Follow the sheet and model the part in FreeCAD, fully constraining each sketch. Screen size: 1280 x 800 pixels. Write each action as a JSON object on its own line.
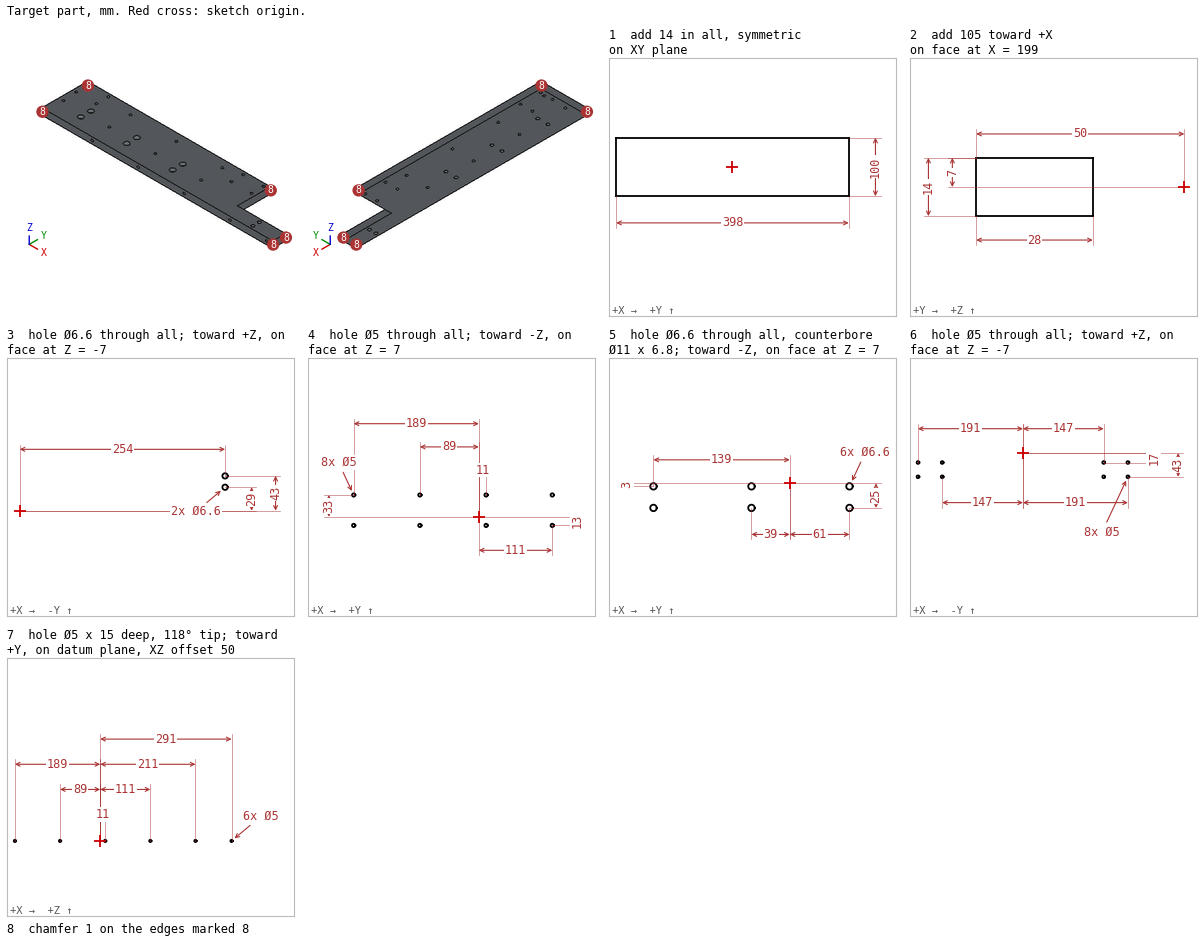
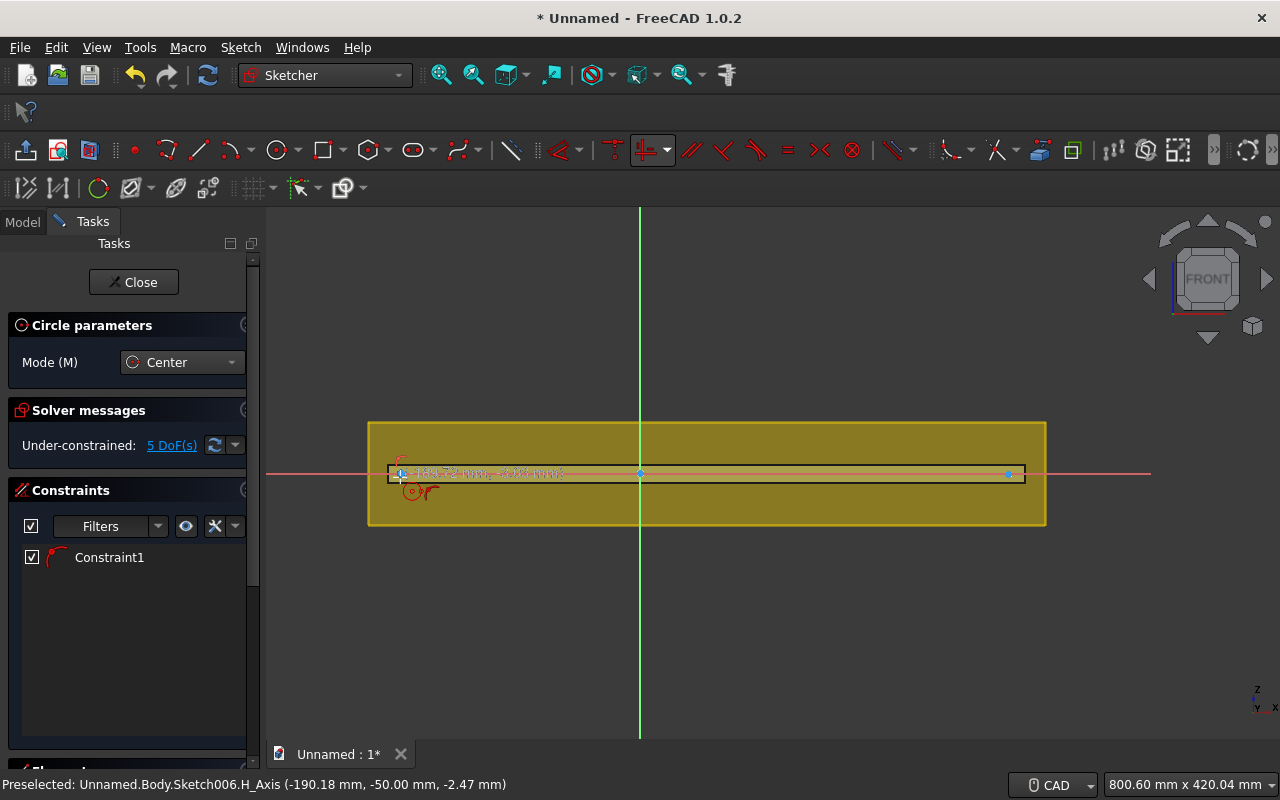
{"action": "scroll", "coordinate": [528, 474], "scroll_direction": "up", "scroll_amount": 10}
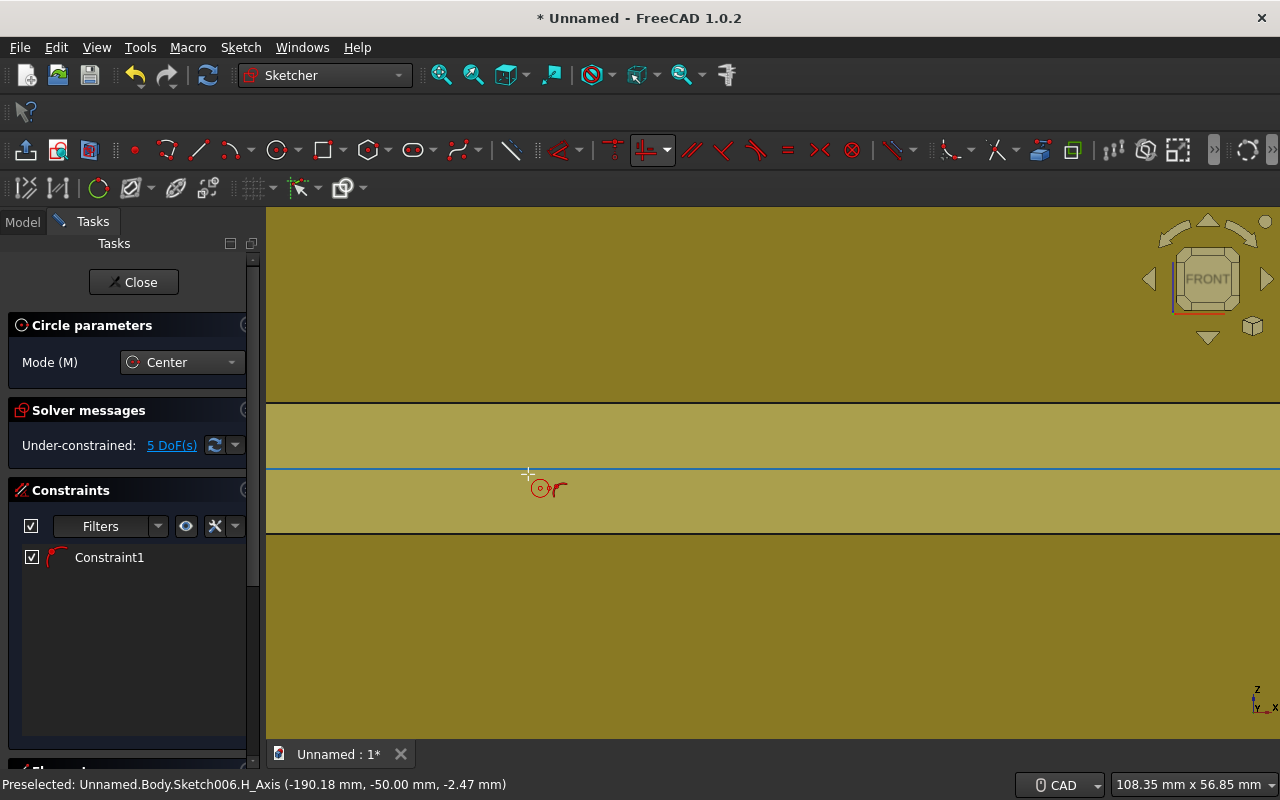
{"action": "scroll", "coordinate": [528, 474], "scroll_direction": "down", "scroll_amount": 10}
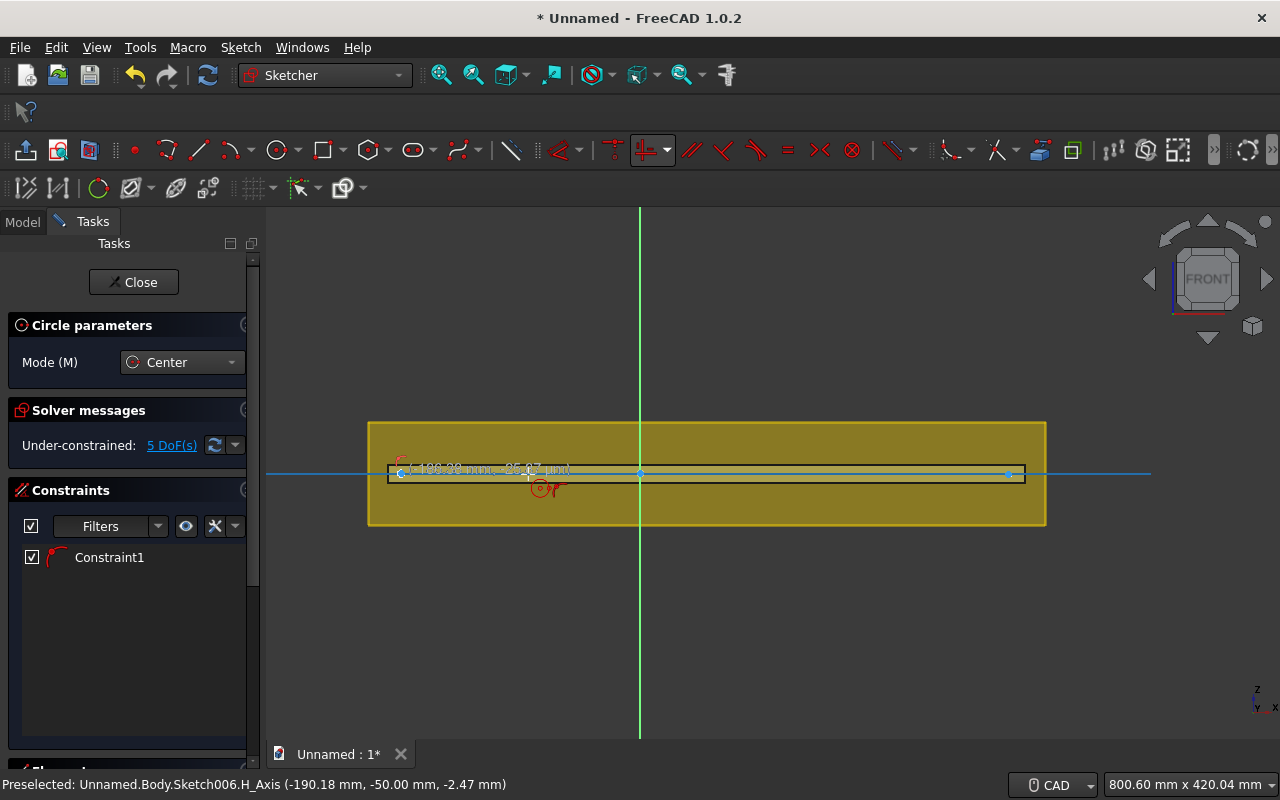
{"action": "left_click", "coordinate": [528, 474]}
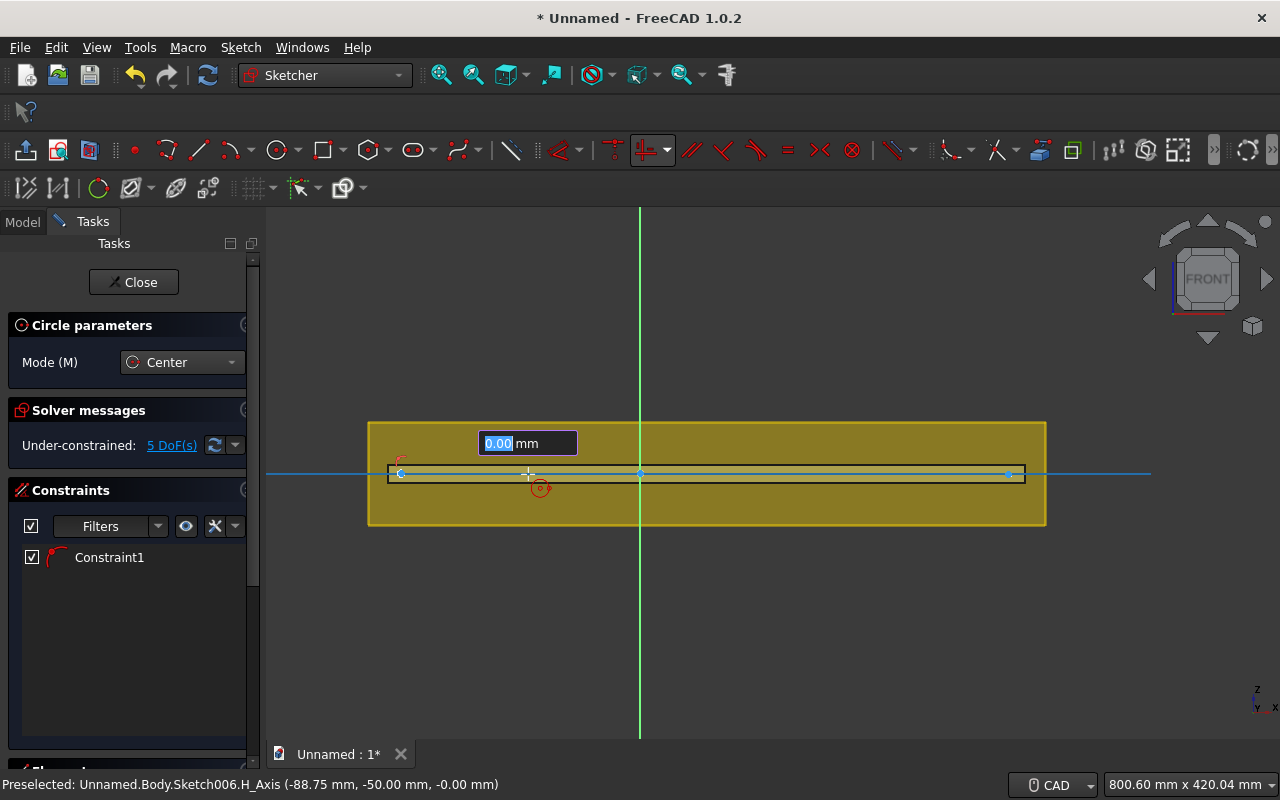
{"action": "scroll", "coordinate": [527, 477], "scroll_direction": "up", "scroll_amount": 9}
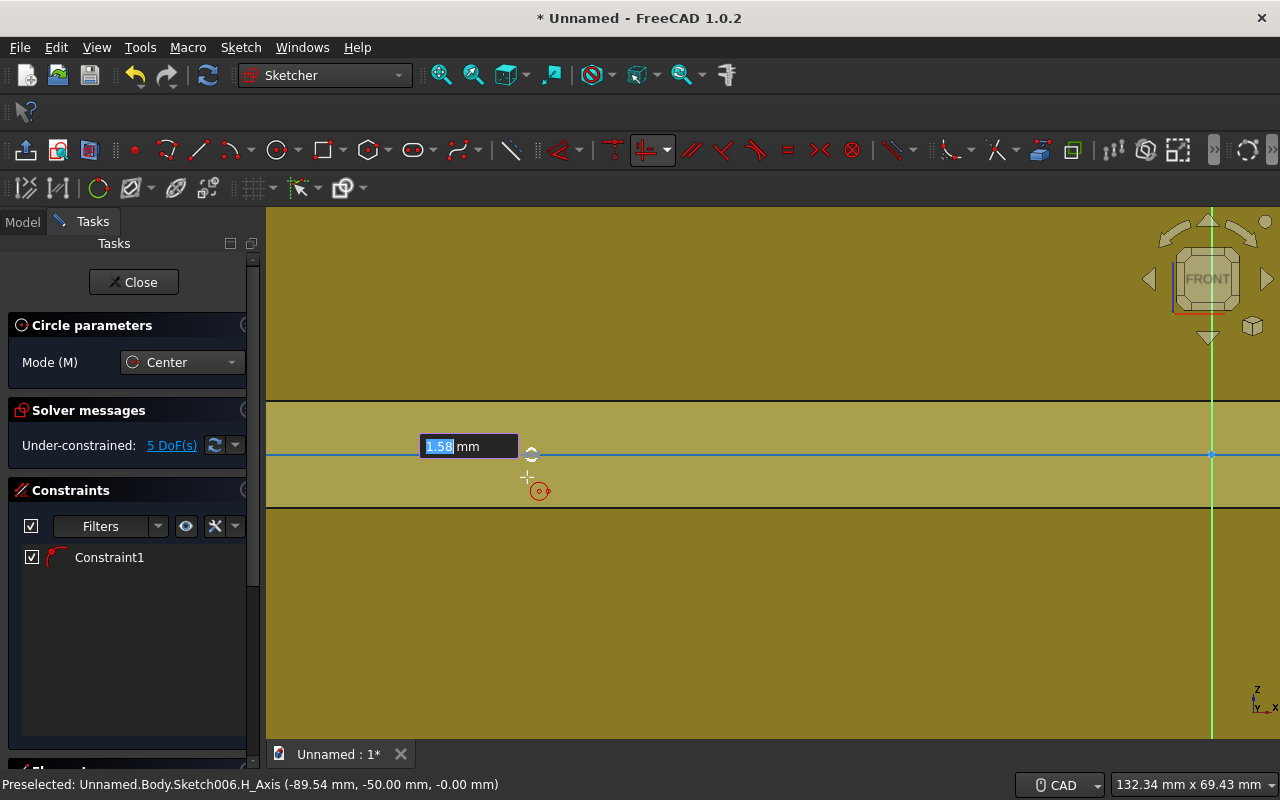
{"action": "left_click", "coordinate": [523, 473]}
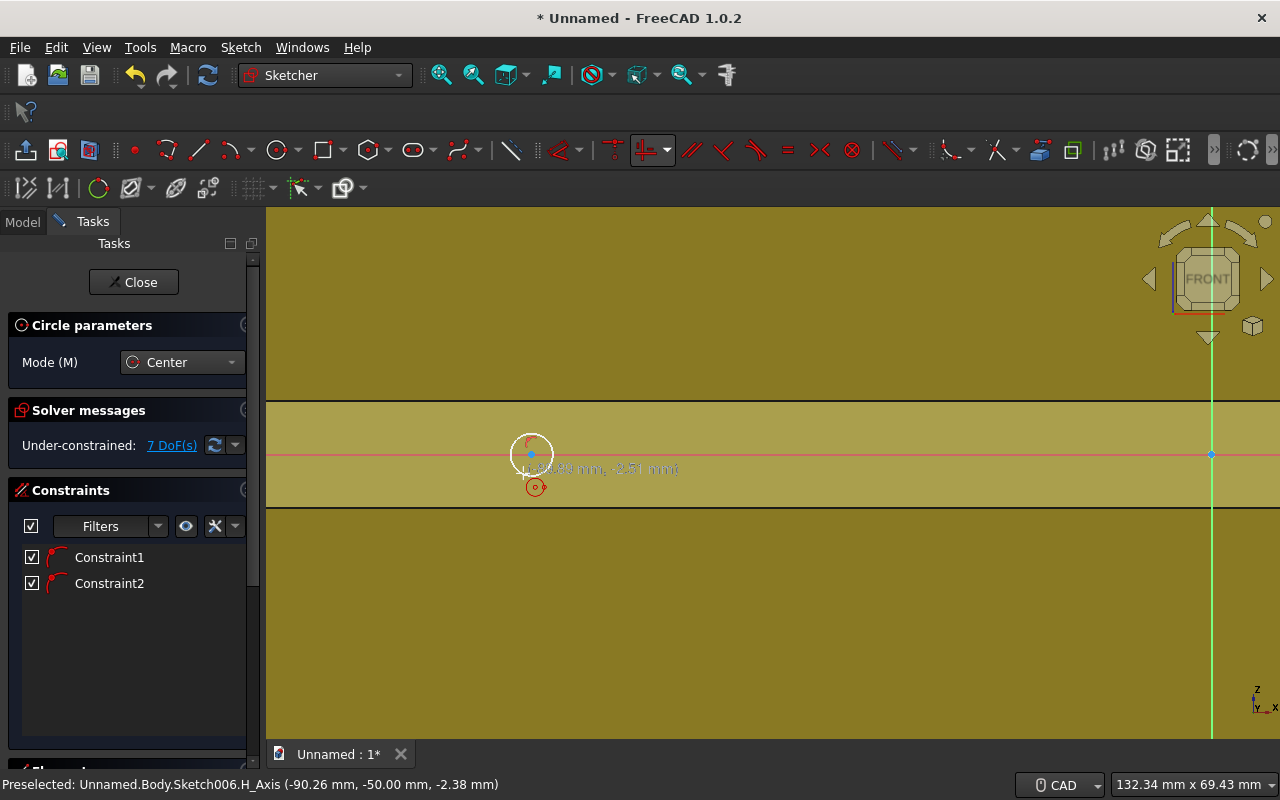
{"action": "scroll", "coordinate": [527, 477], "scroll_direction": "down", "scroll_amount": 9}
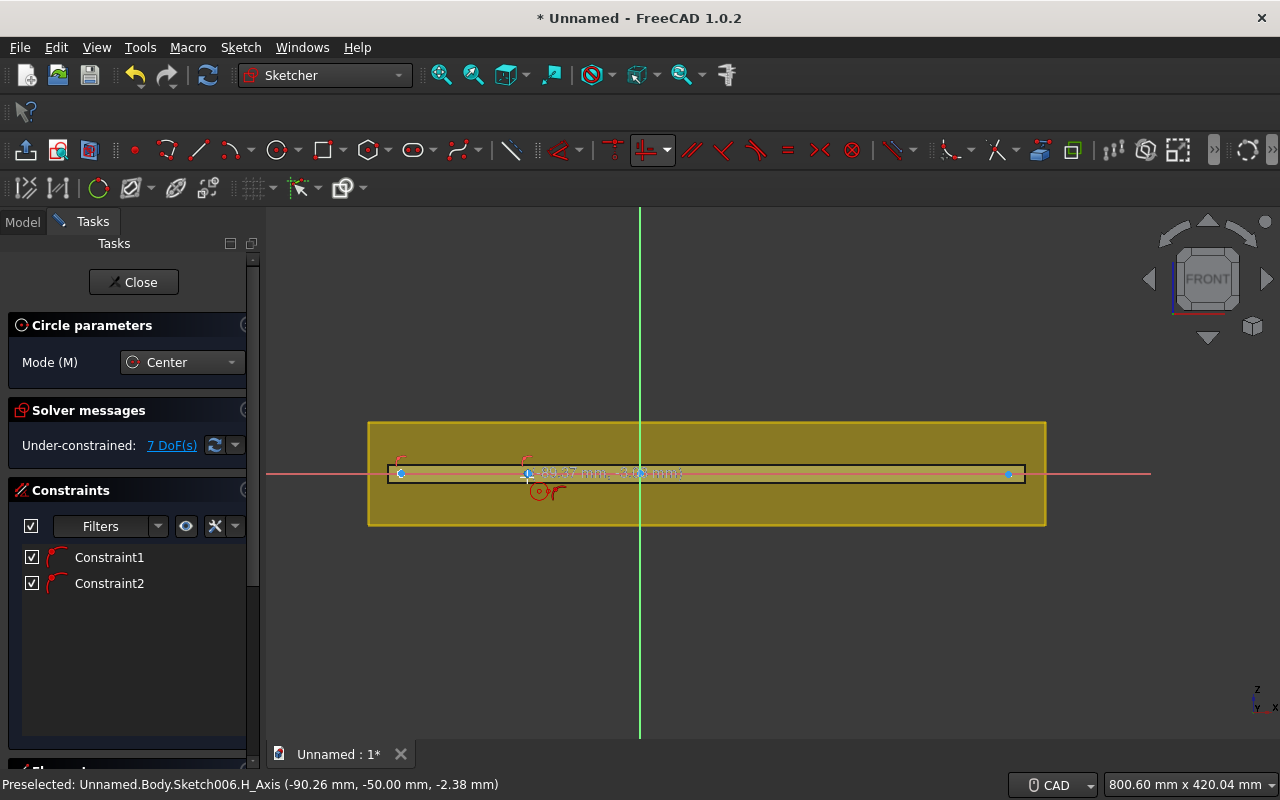
{"action": "scroll", "coordinate": [654, 474], "scroll_direction": "up", "scroll_amount": 10}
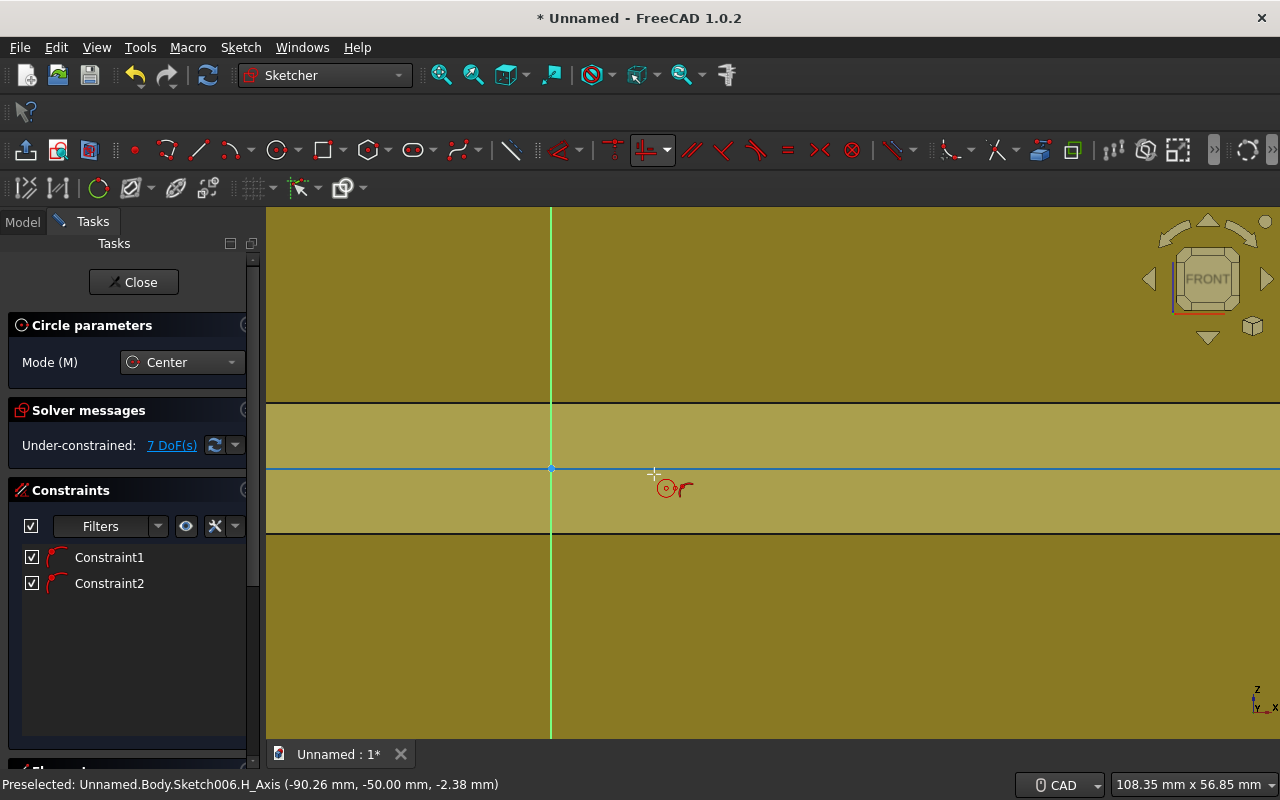
{"action": "scroll", "coordinate": [654, 474], "scroll_direction": "down", "scroll_amount": 10}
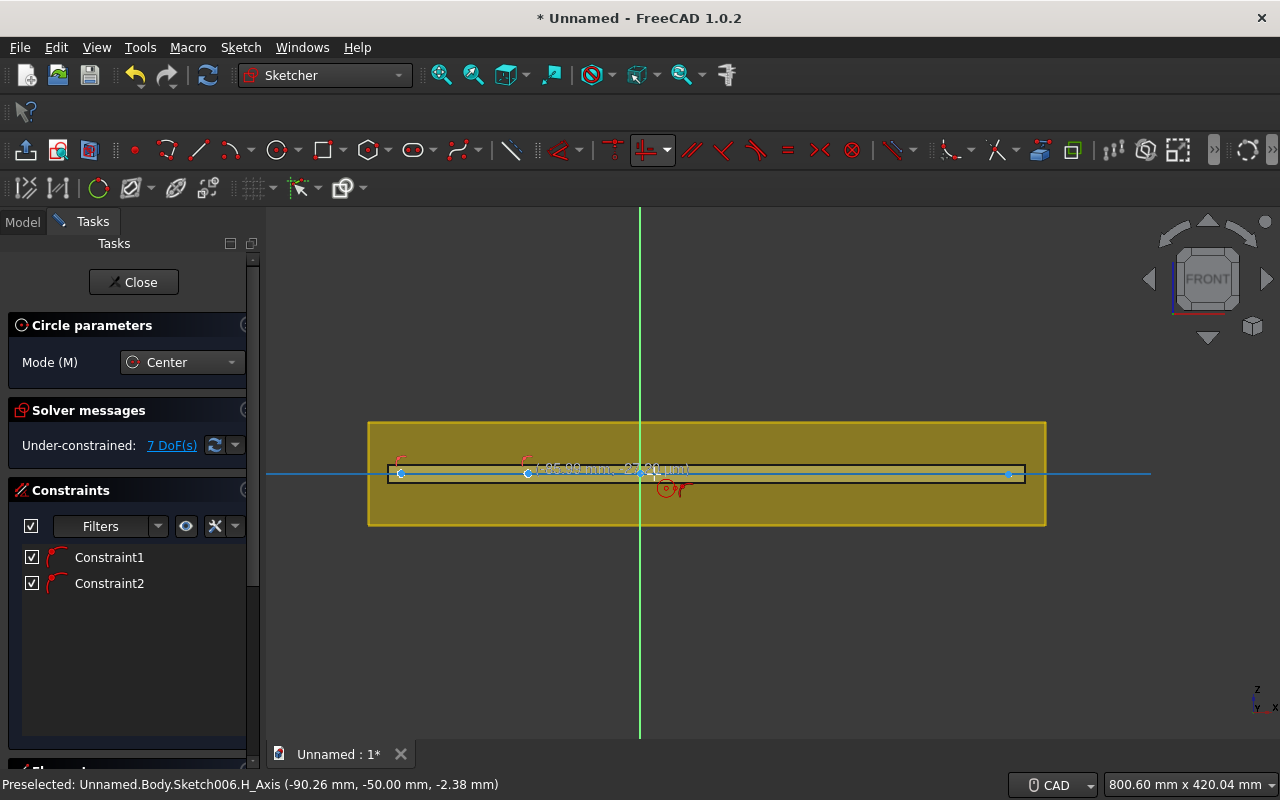
{"action": "left_click", "coordinate": [654, 474]}